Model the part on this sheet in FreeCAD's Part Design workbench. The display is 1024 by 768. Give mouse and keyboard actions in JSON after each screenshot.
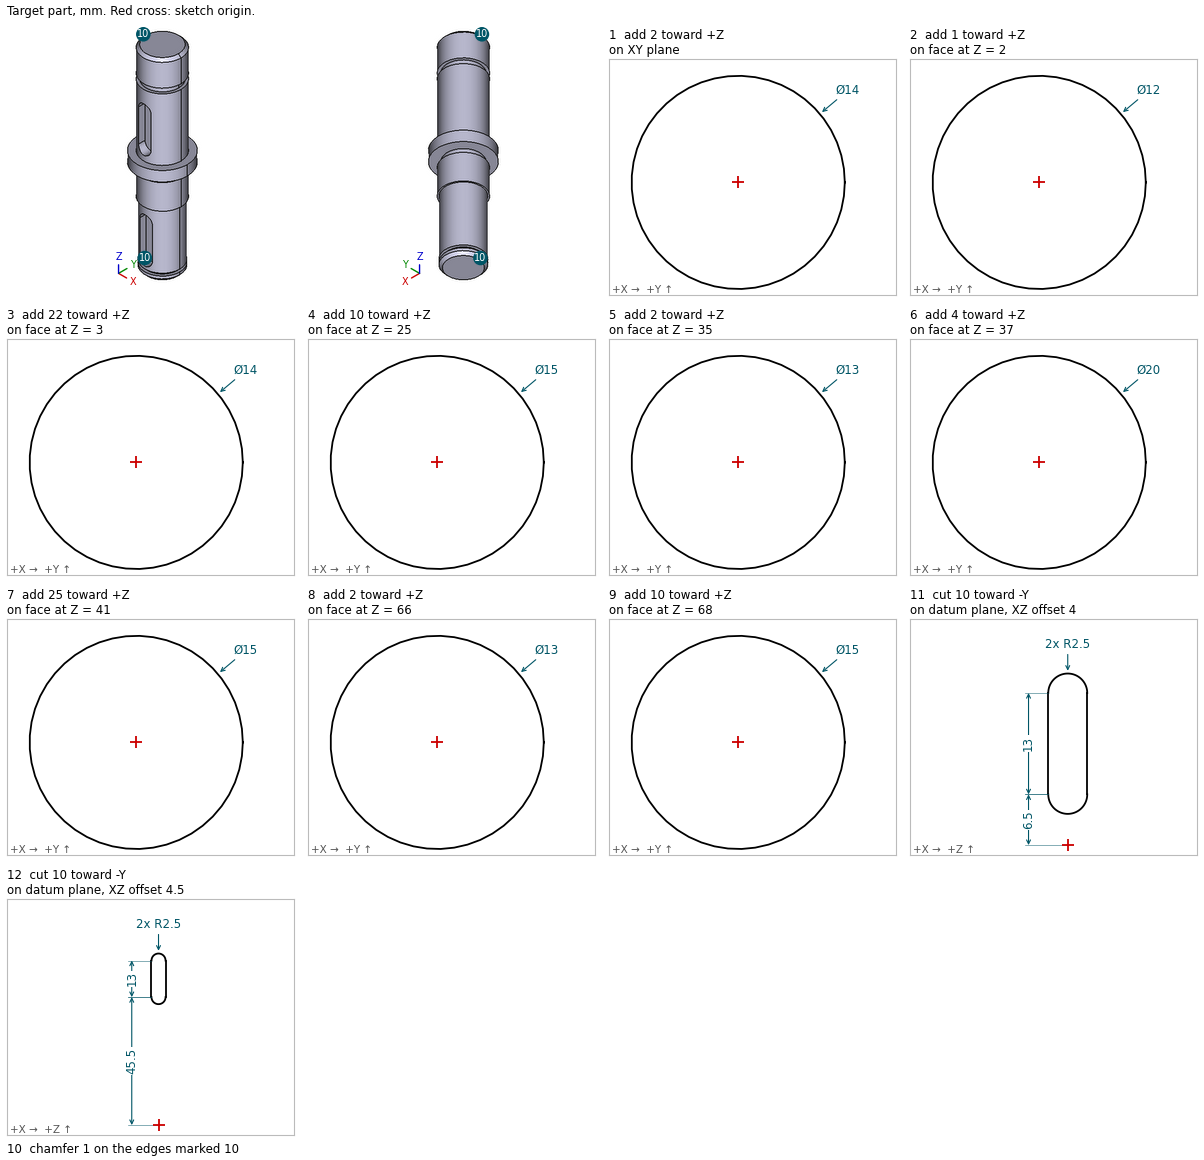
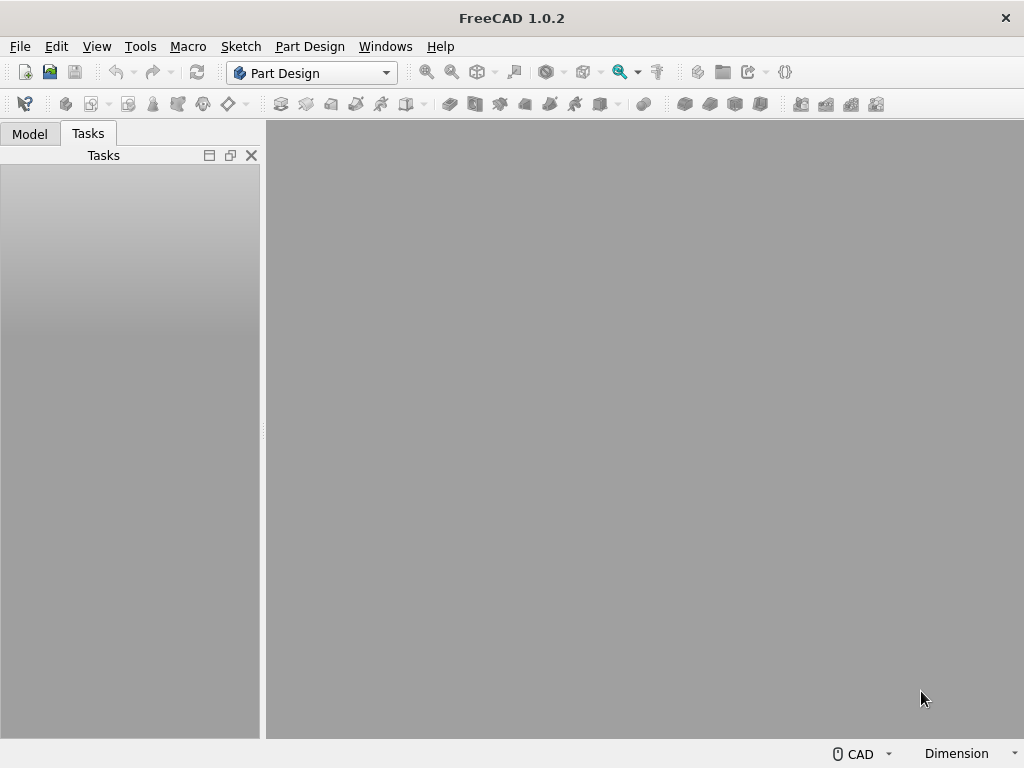
{"action": "left_click", "coordinate": [25, 72]}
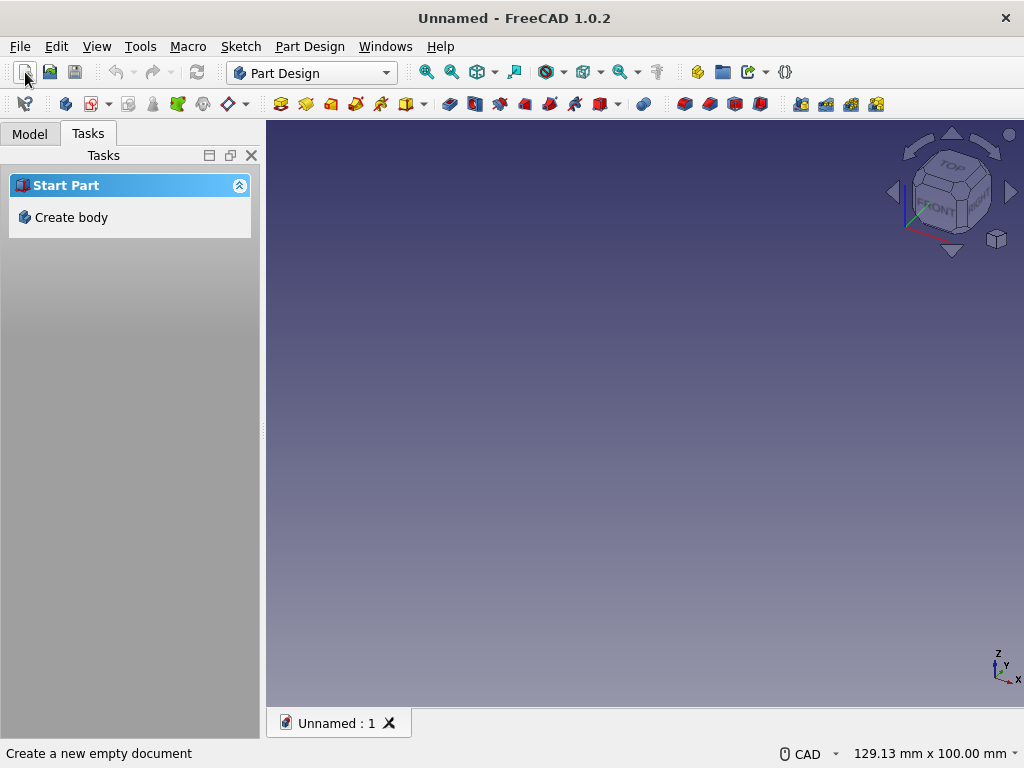
{"action": "left_click", "coordinate": [90, 104]}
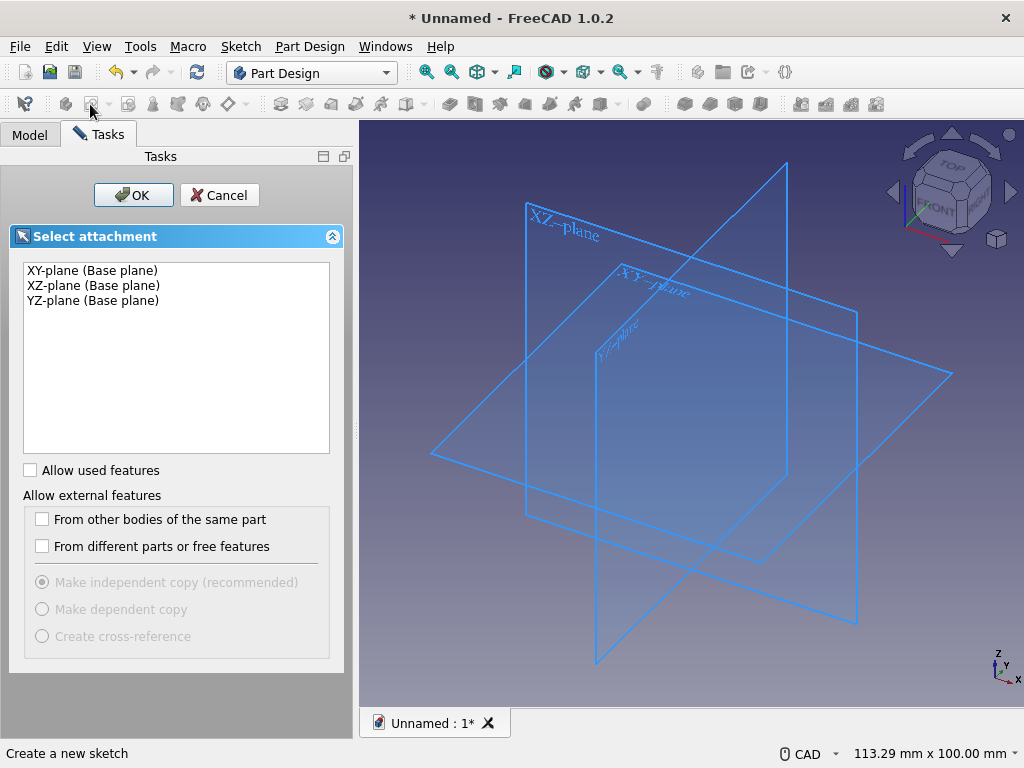
{"action": "left_click", "coordinate": [84, 270]}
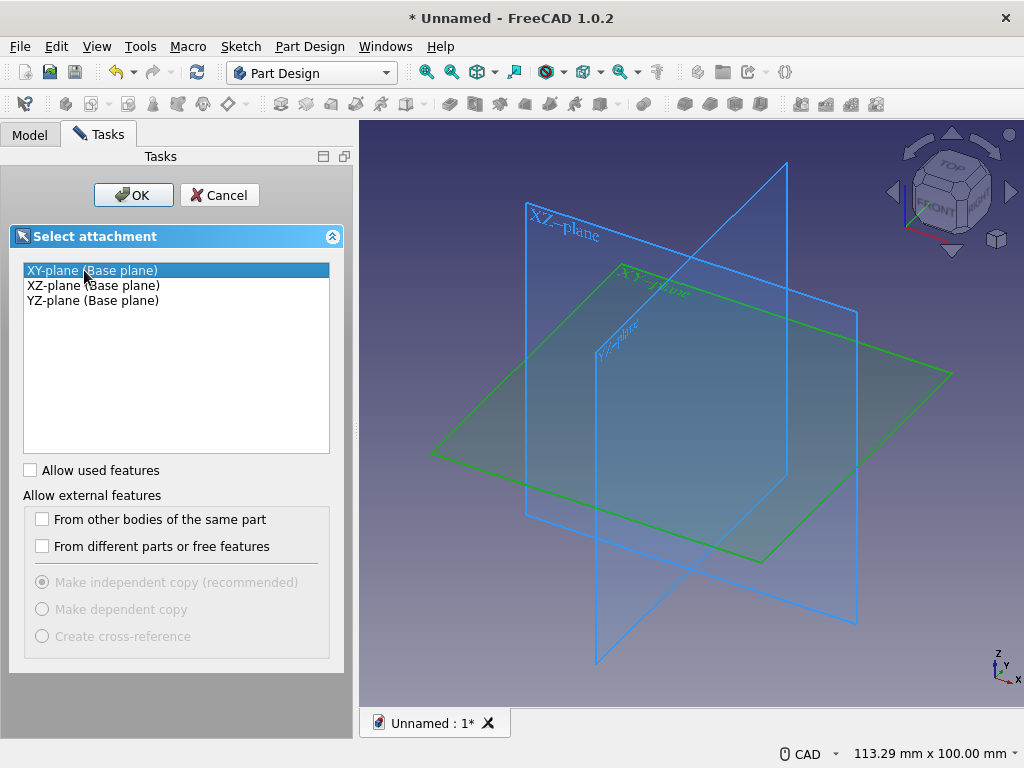
{"action": "left_click", "coordinate": [134, 195]}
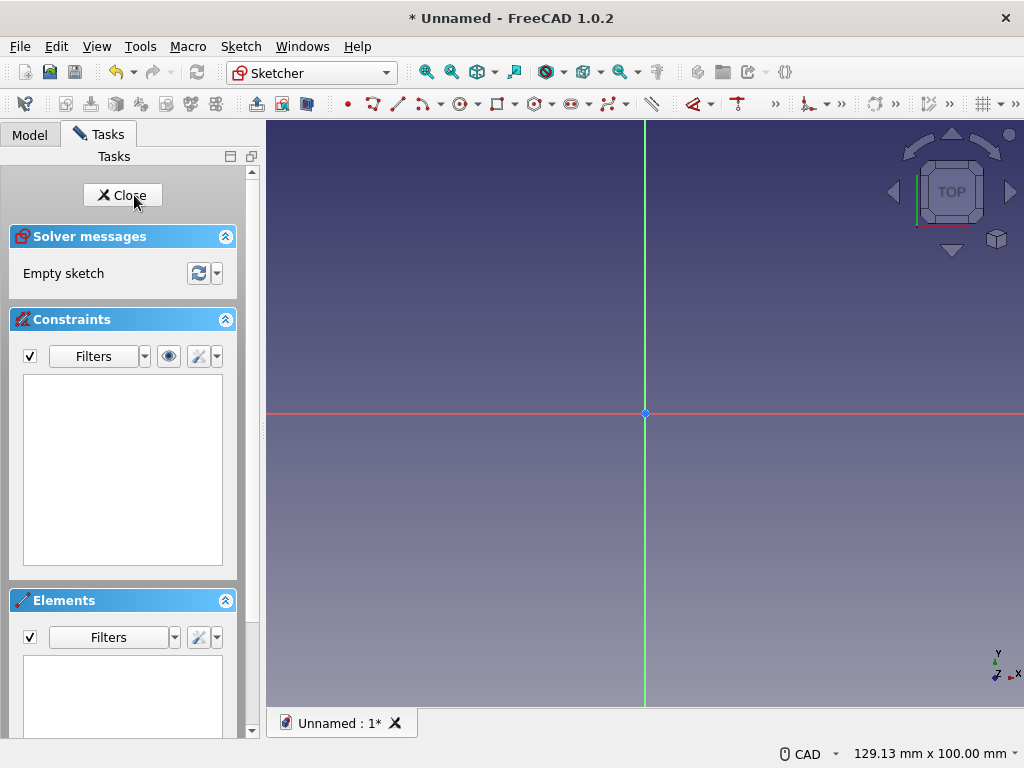
{"action": "scroll", "coordinate": [662, 414], "scroll_direction": "up", "scroll_amount": 8}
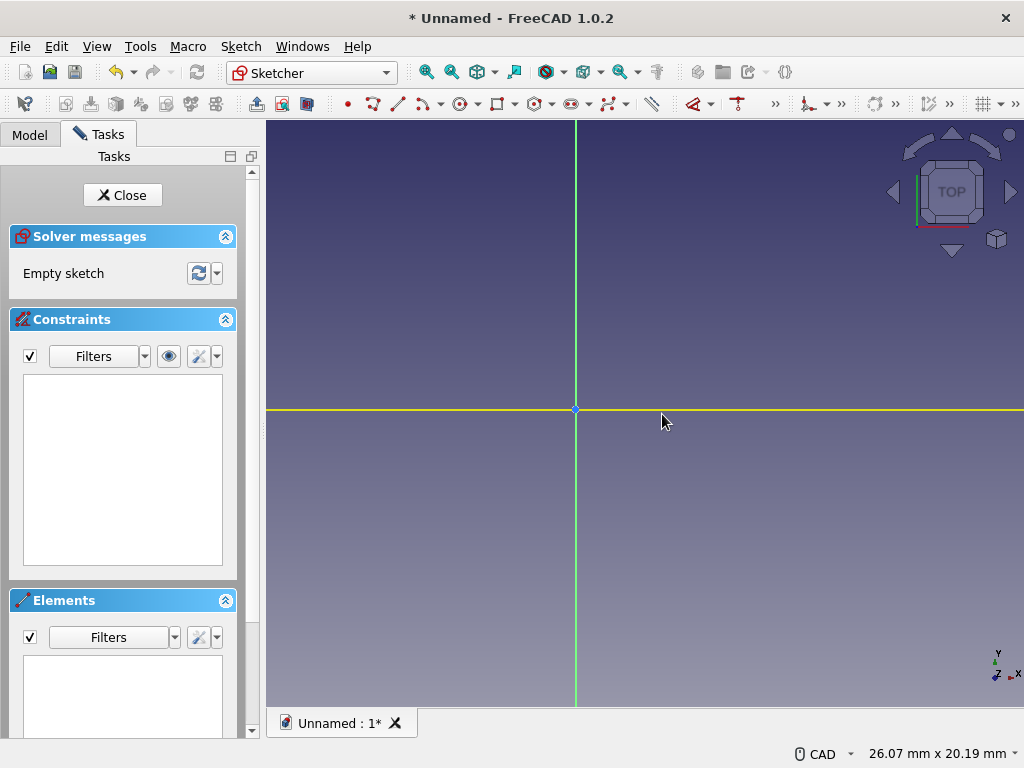
{"action": "left_click", "coordinate": [460, 104]}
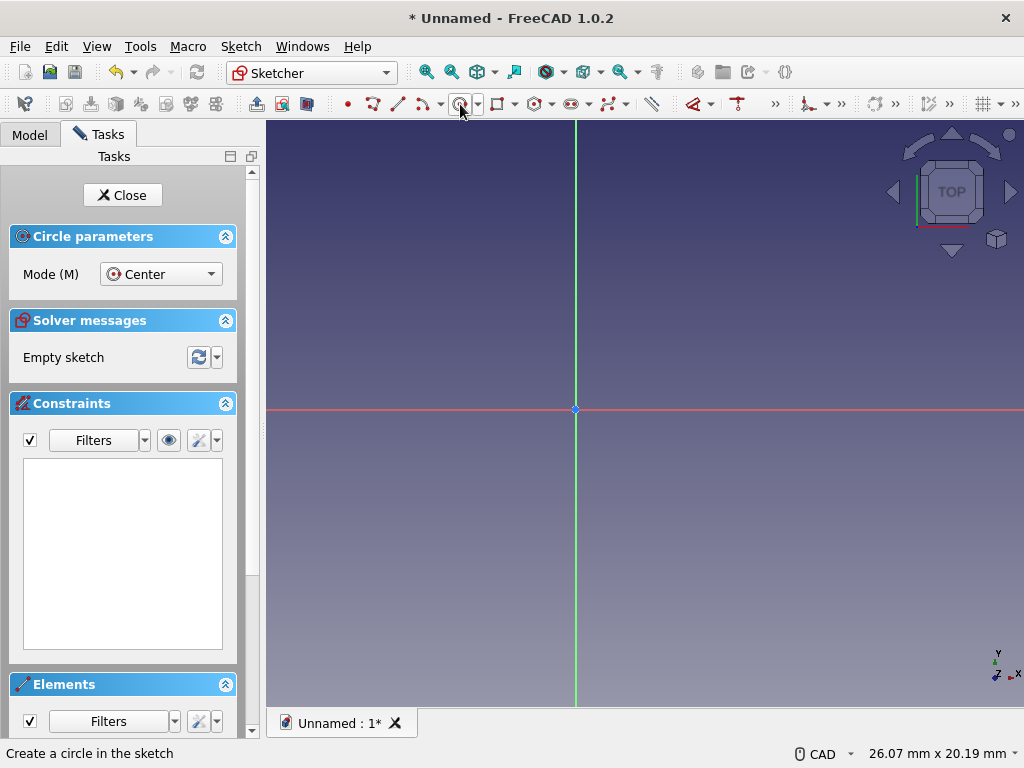
{"action": "left_click", "coordinate": [576, 410]}
{"action": "left_click", "coordinate": [720, 266]}
{"action": "key", "text": "Escape"}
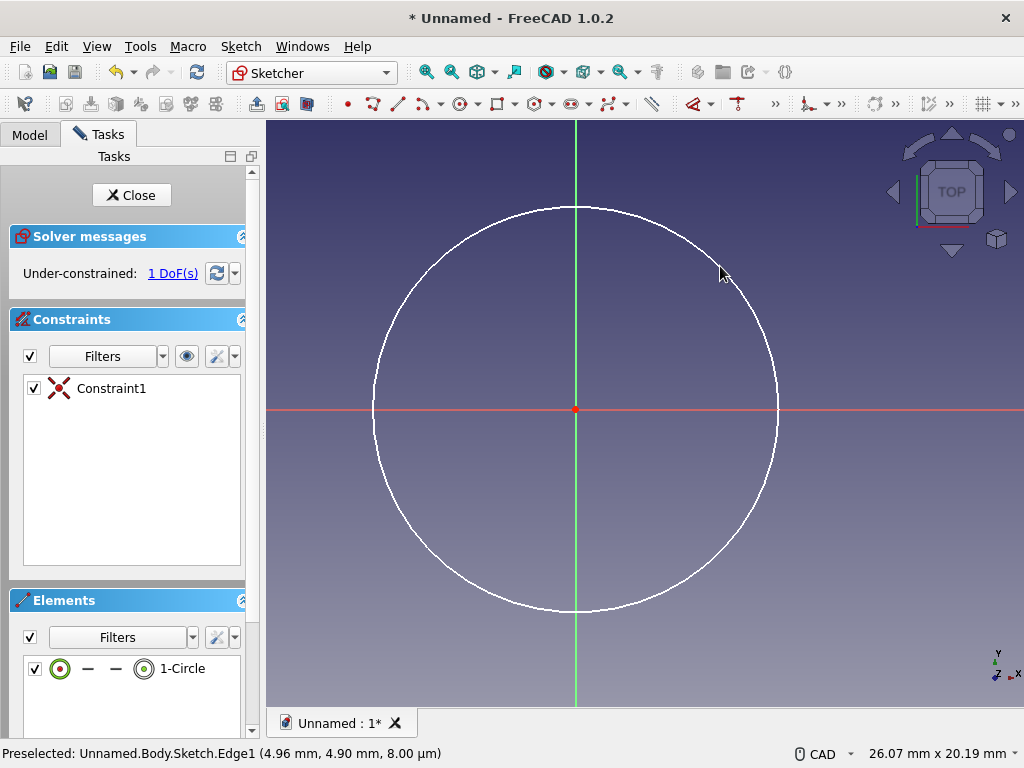
{"action": "left_click", "coordinate": [692, 104]}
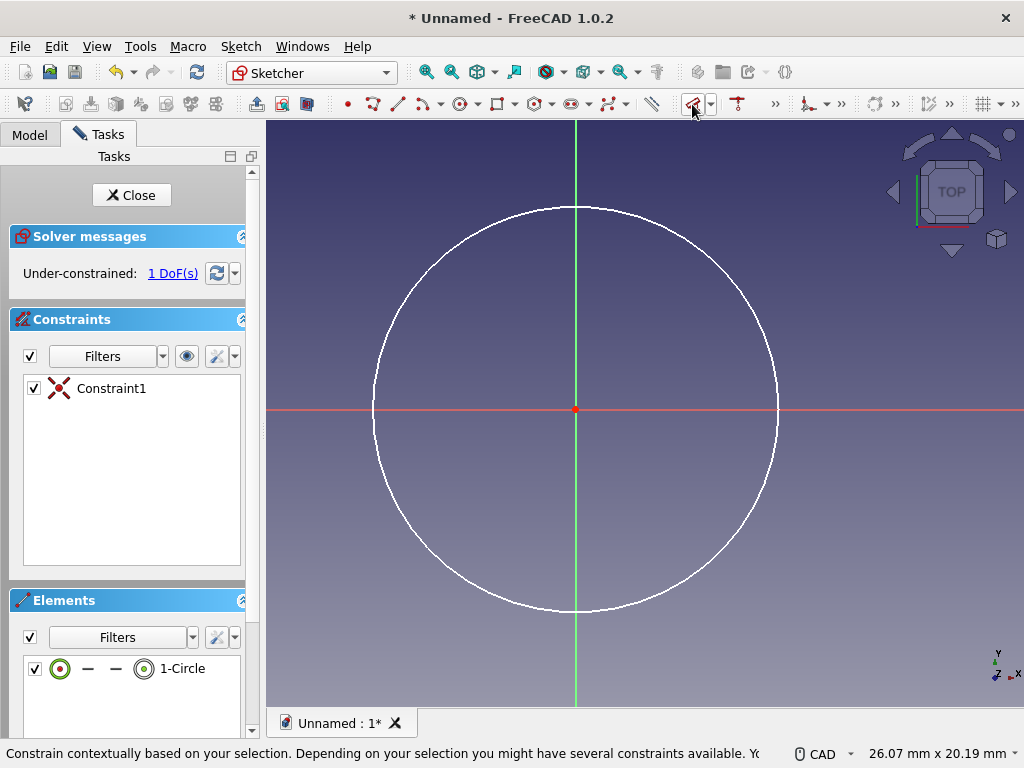
{"action": "left_click", "coordinate": [719, 266]}
{"action": "left_click", "coordinate": [742, 243]}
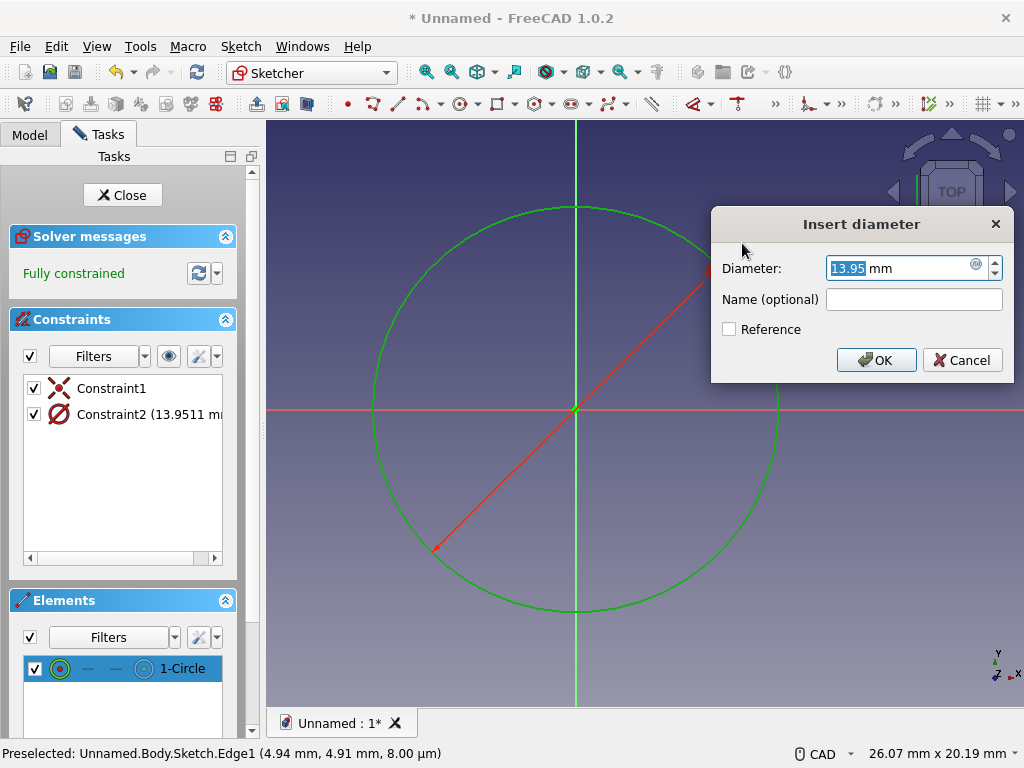
{"action": "type", "text": "14"}
{"action": "key", "text": "Return"}
{"action": "key", "text": "Escape"}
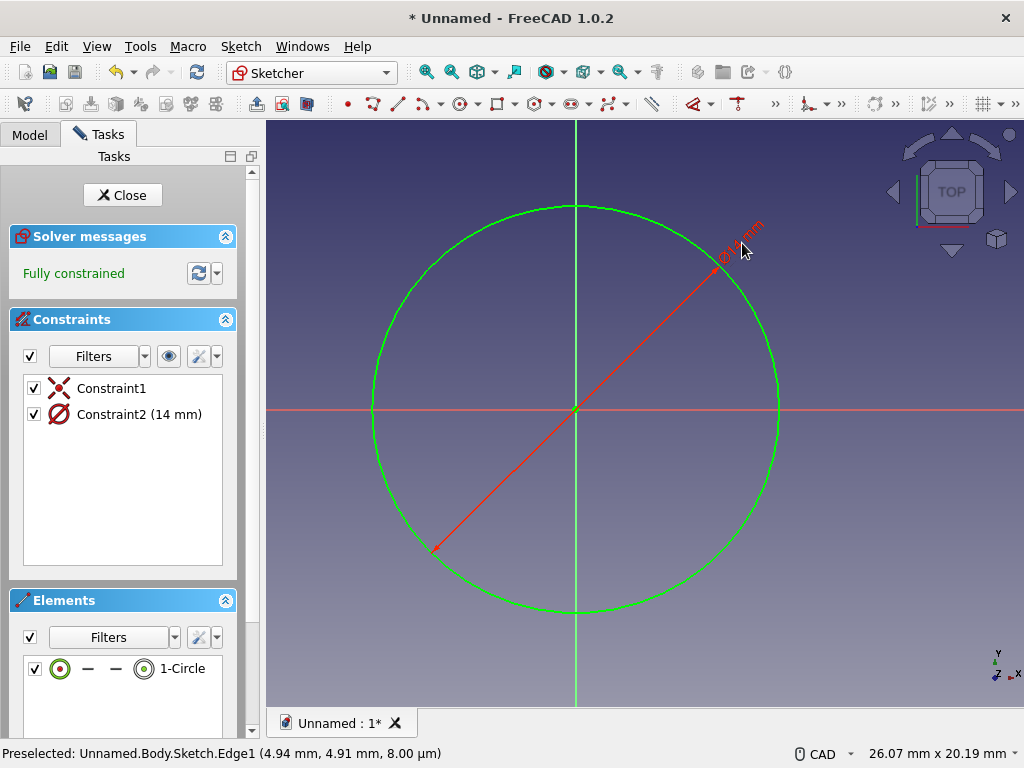
{"action": "left_click", "coordinate": [123, 195]}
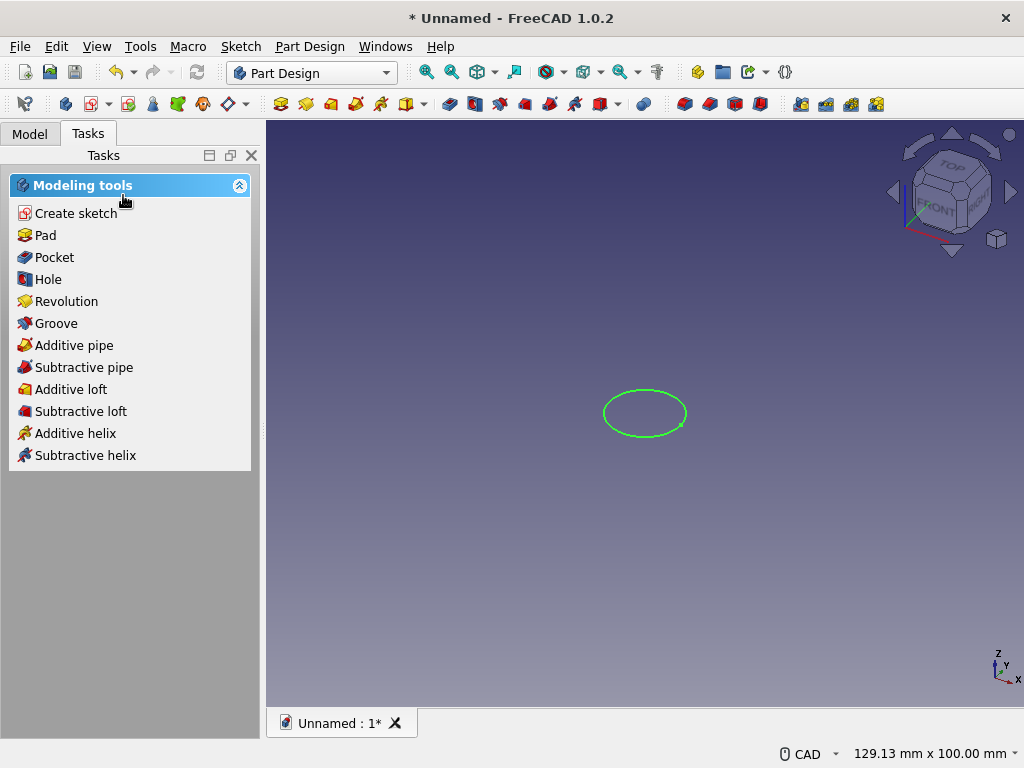
{"action": "left_click", "coordinate": [281, 104]}